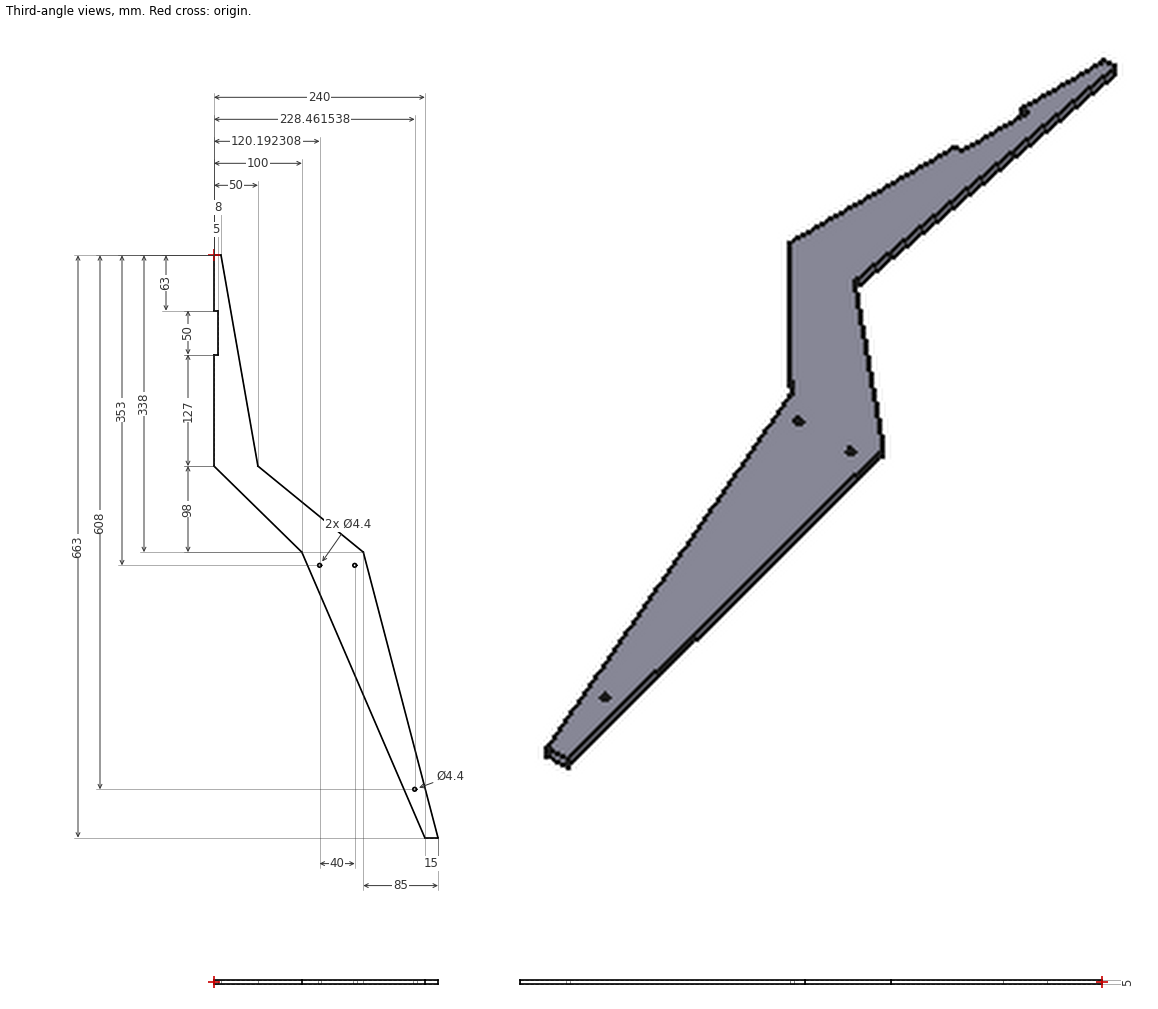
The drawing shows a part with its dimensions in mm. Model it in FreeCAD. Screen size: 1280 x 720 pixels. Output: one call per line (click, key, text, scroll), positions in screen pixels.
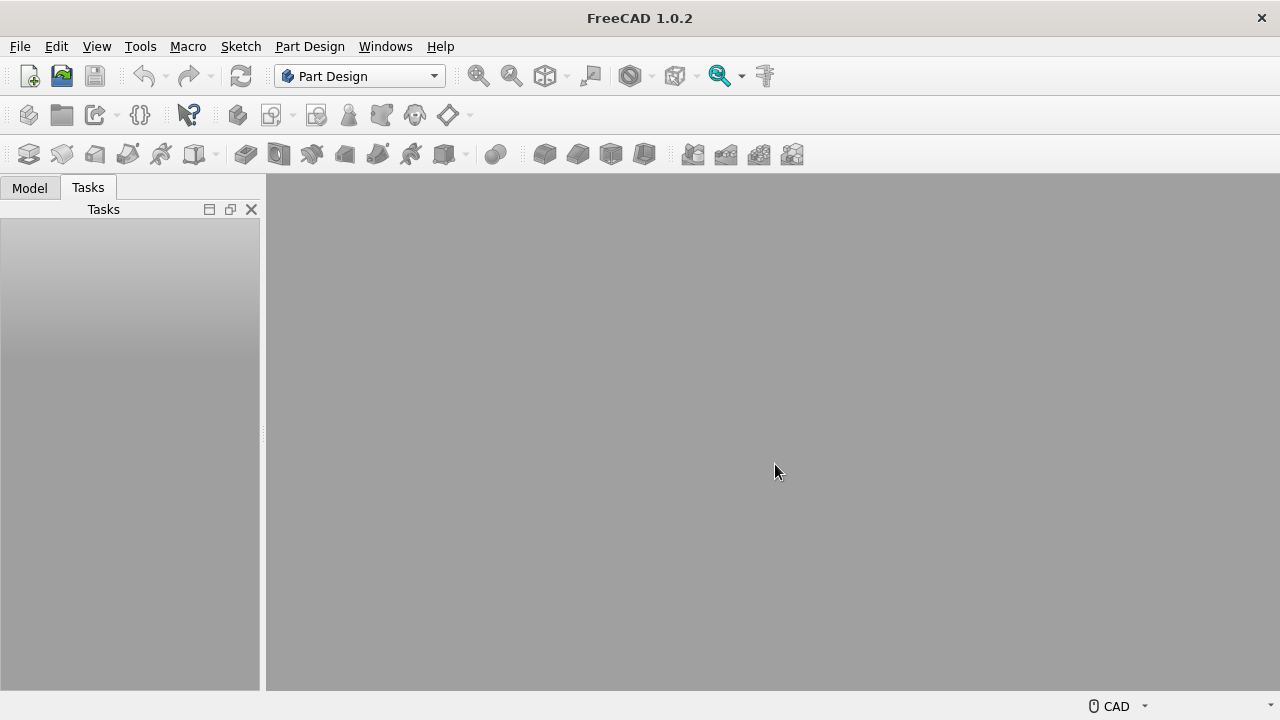
click(29, 76)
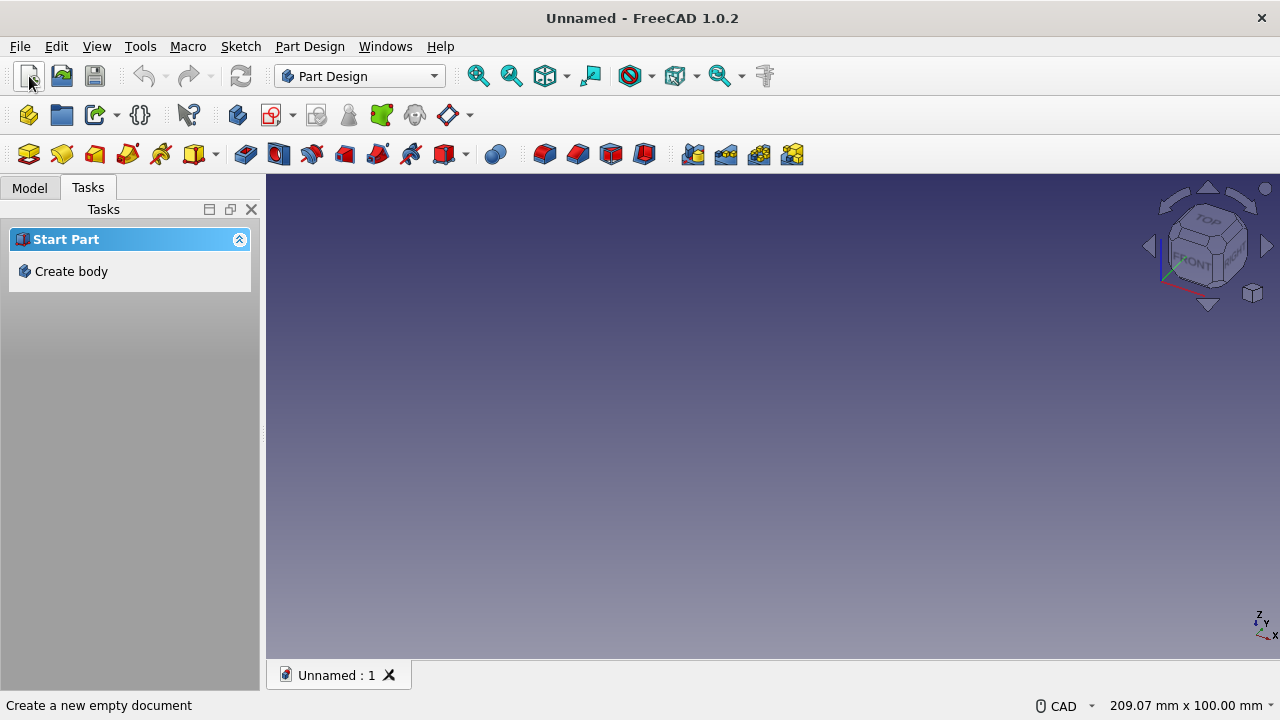
click(270, 116)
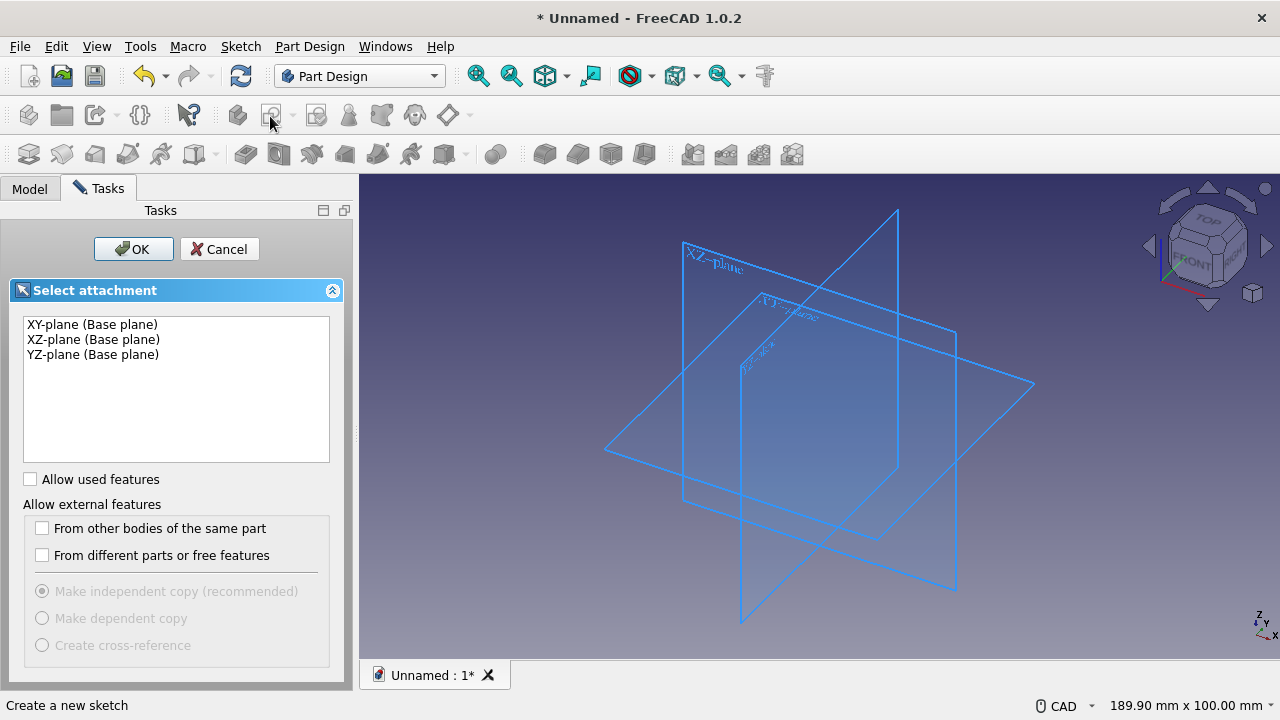
click(84, 324)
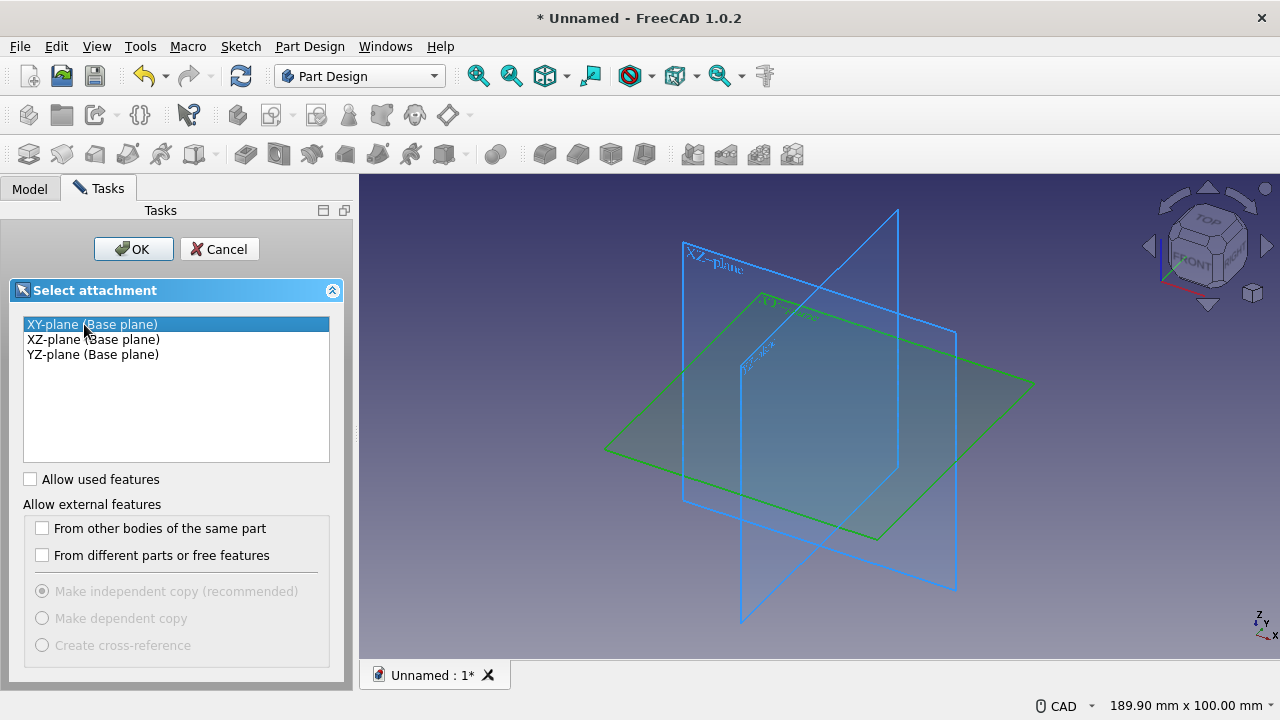
click(134, 249)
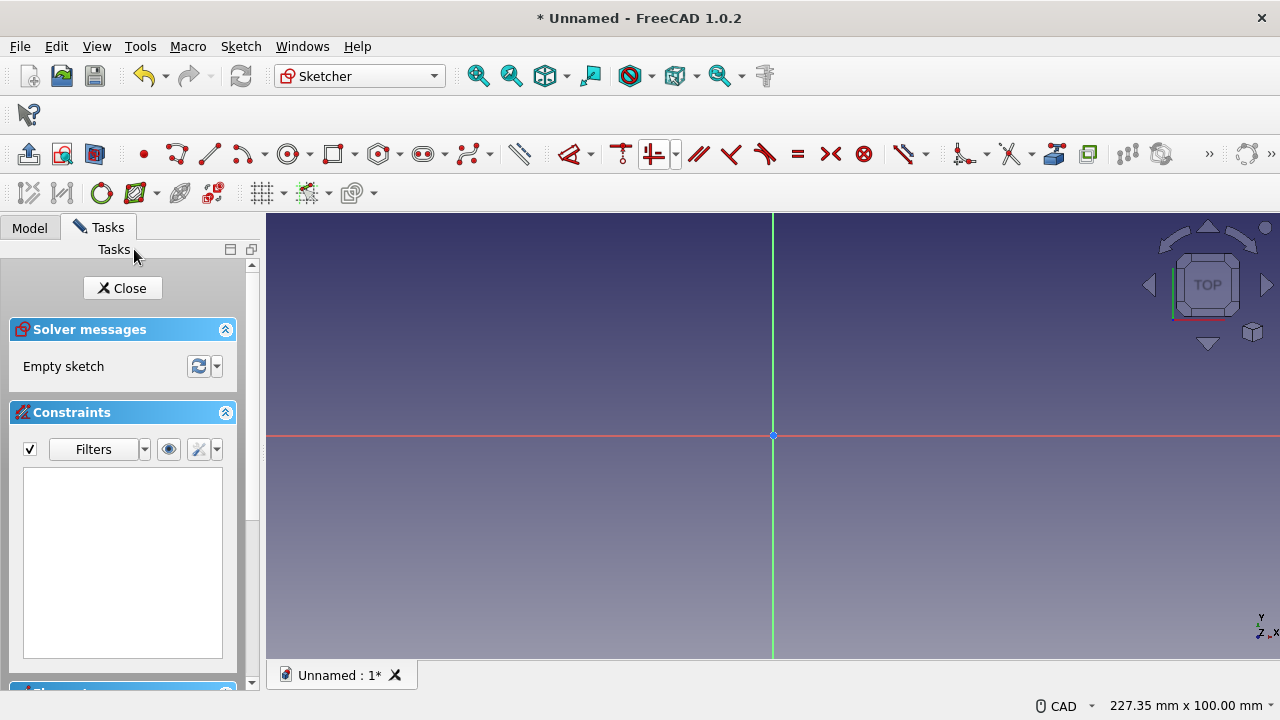
scroll(641, 288, down, 12)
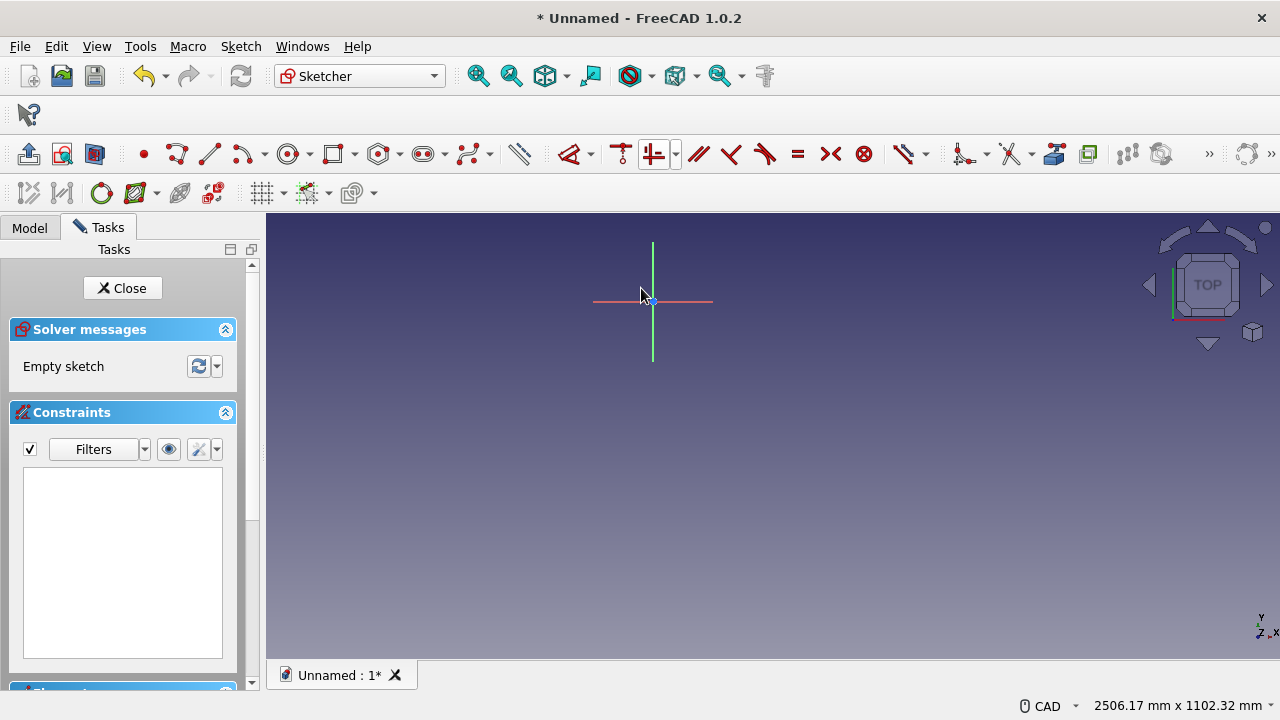
click(177, 154)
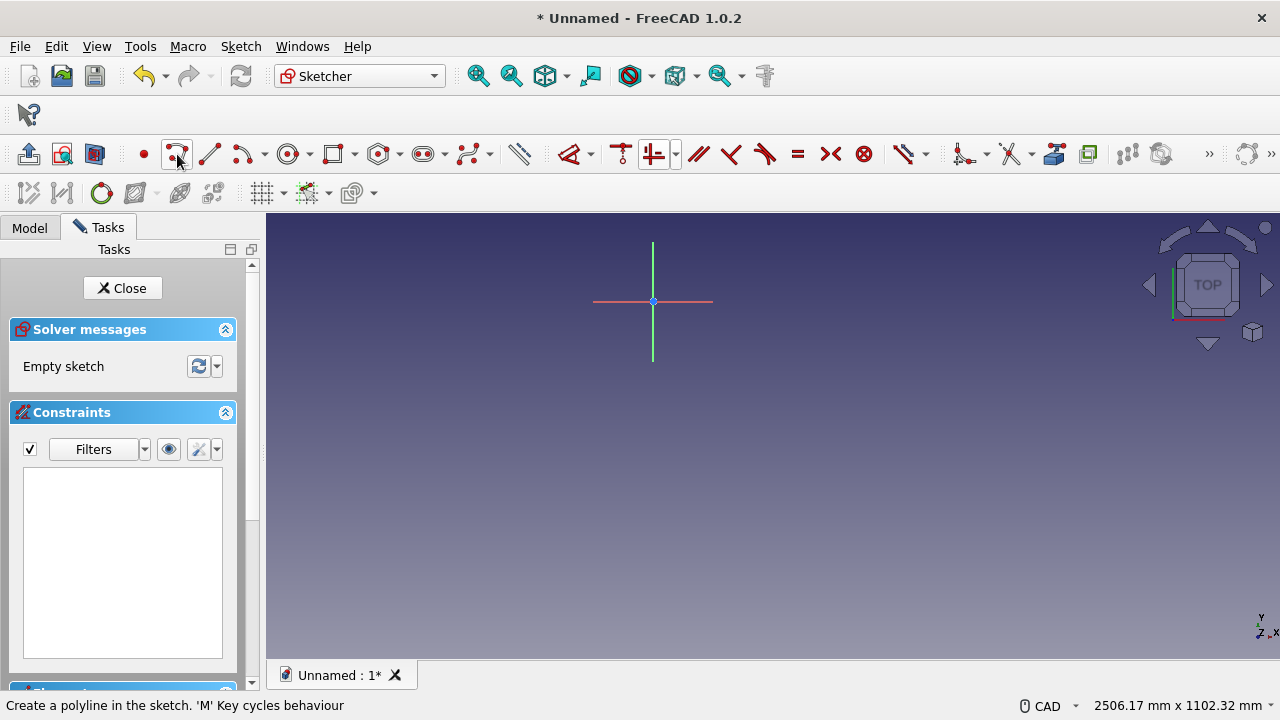
click(653, 302)
click(662, 327)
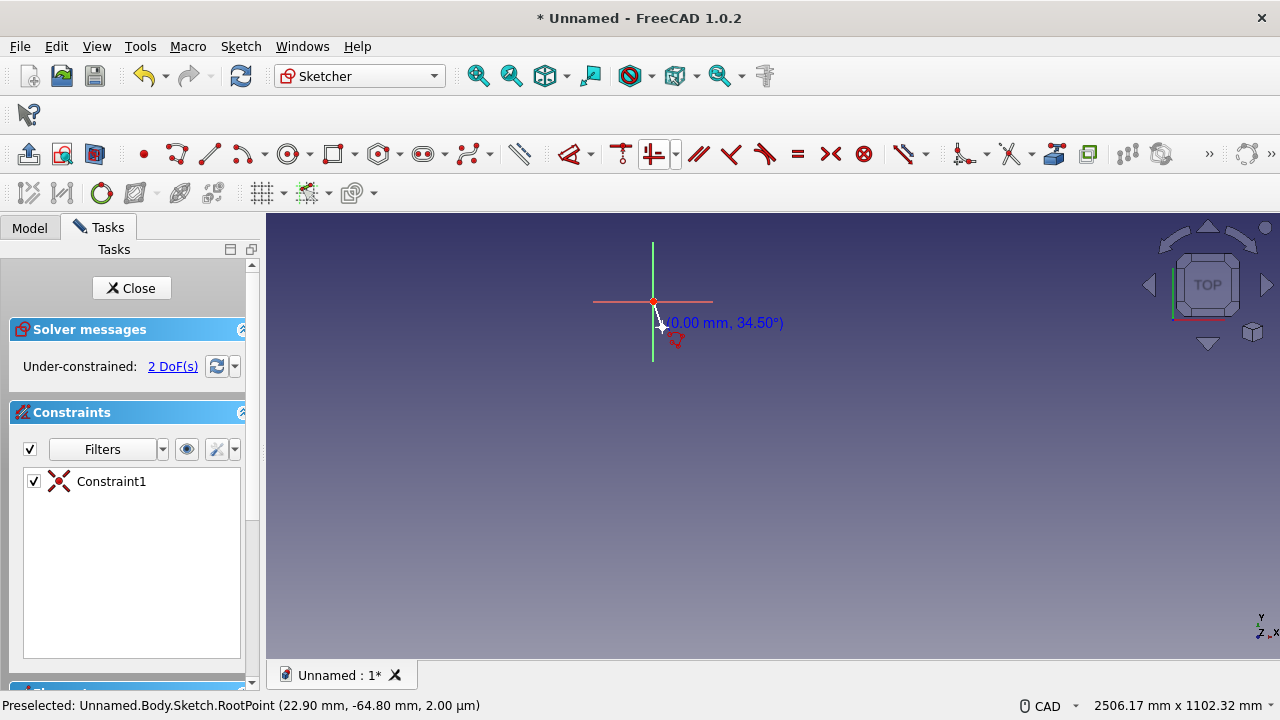
scroll(655, 327, up, 11)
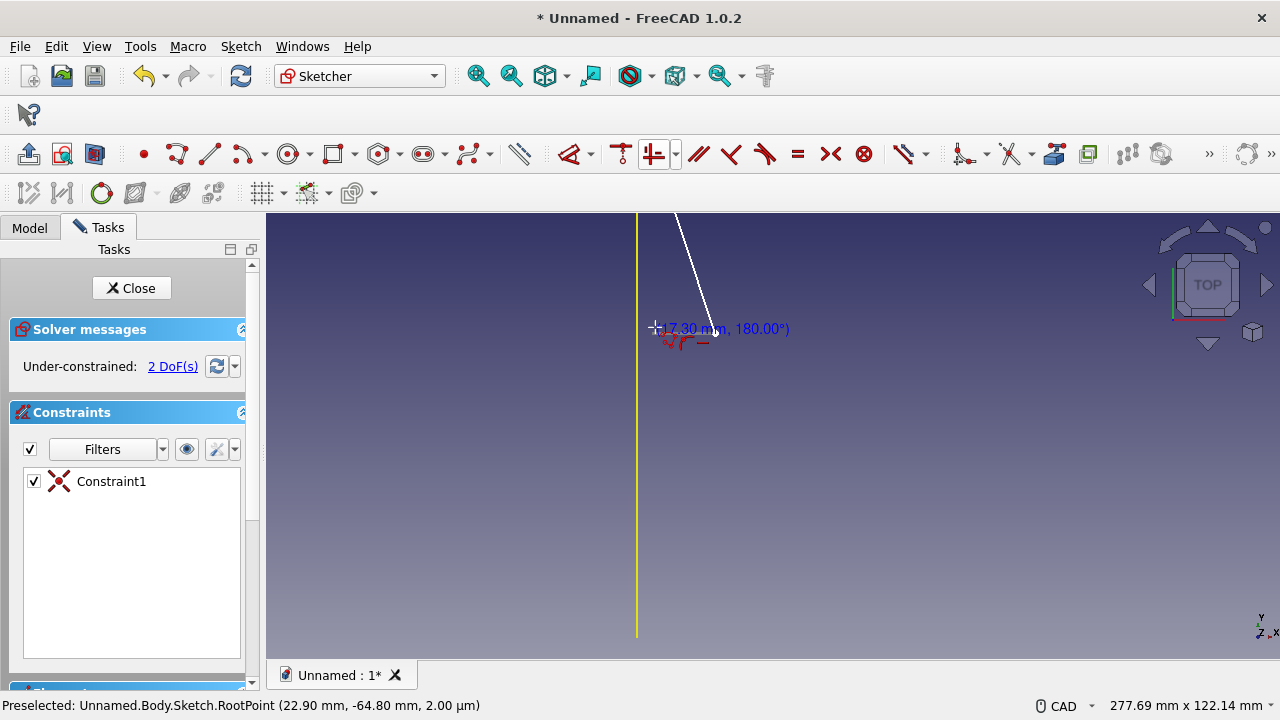
click(655, 325)
click(655, 508)
click(637, 508)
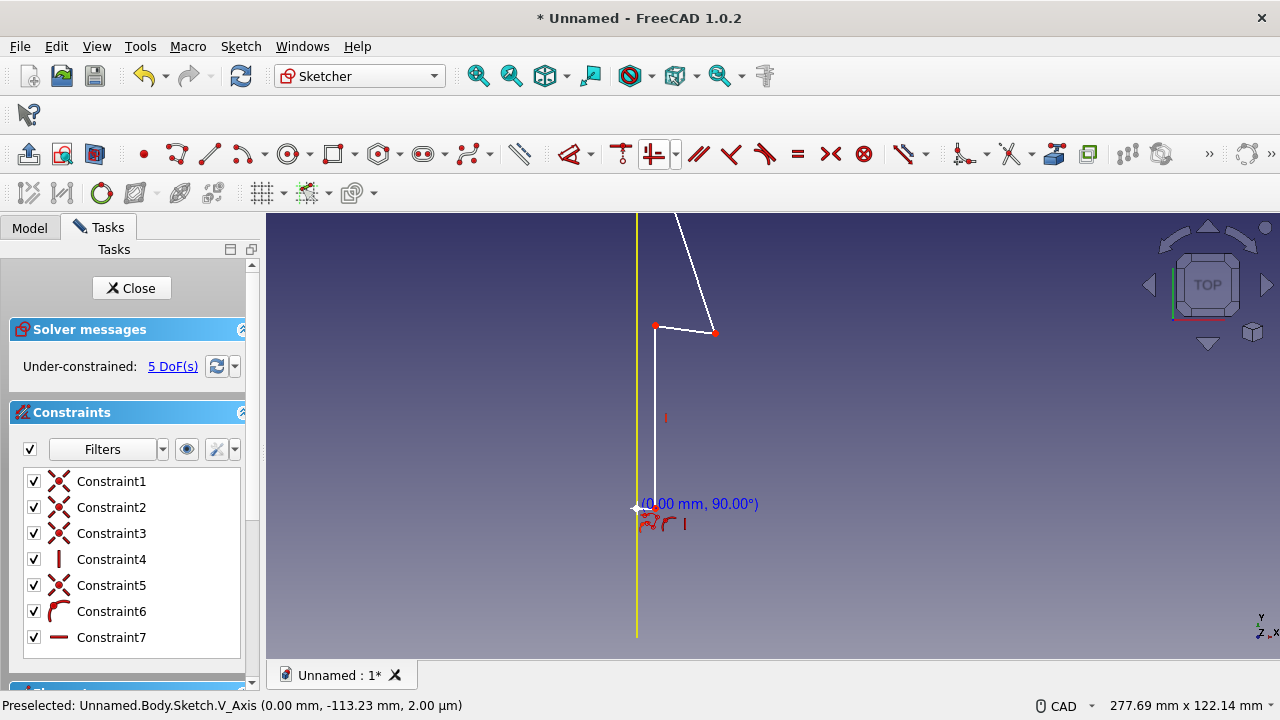
scroll(655, 328, down, 11)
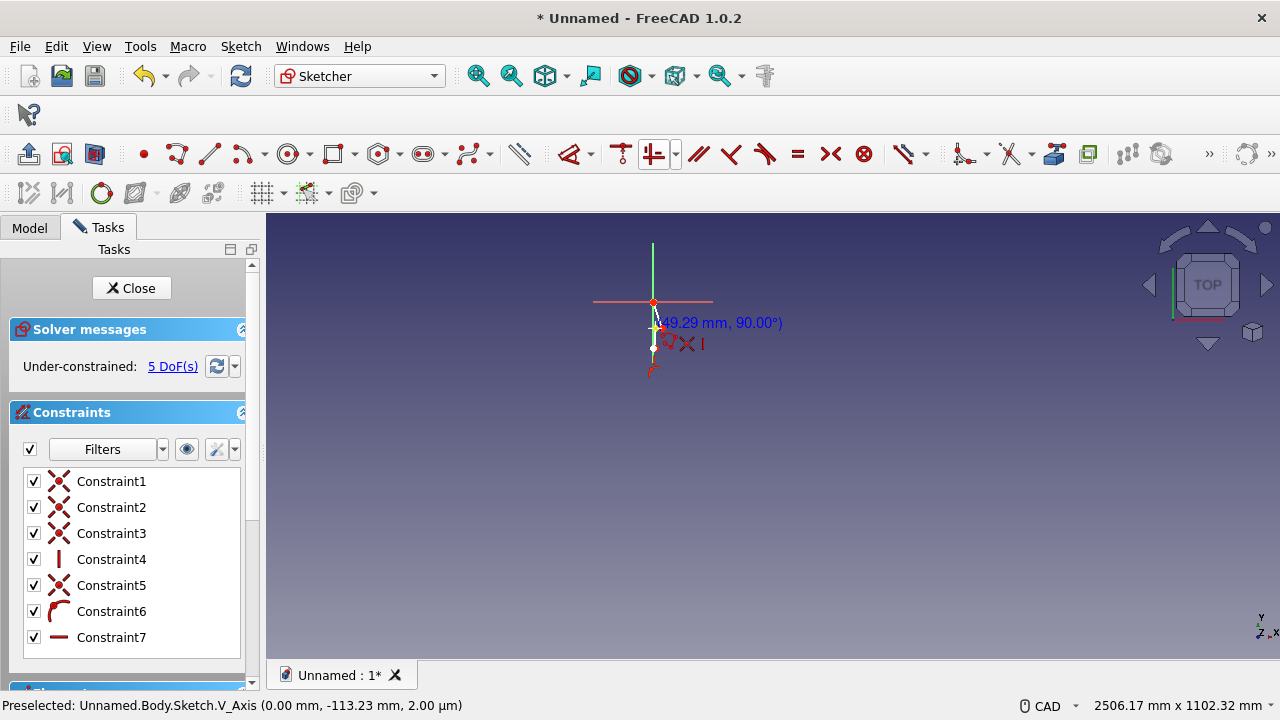
click(662, 400)
click(694, 439)
click(750, 571)